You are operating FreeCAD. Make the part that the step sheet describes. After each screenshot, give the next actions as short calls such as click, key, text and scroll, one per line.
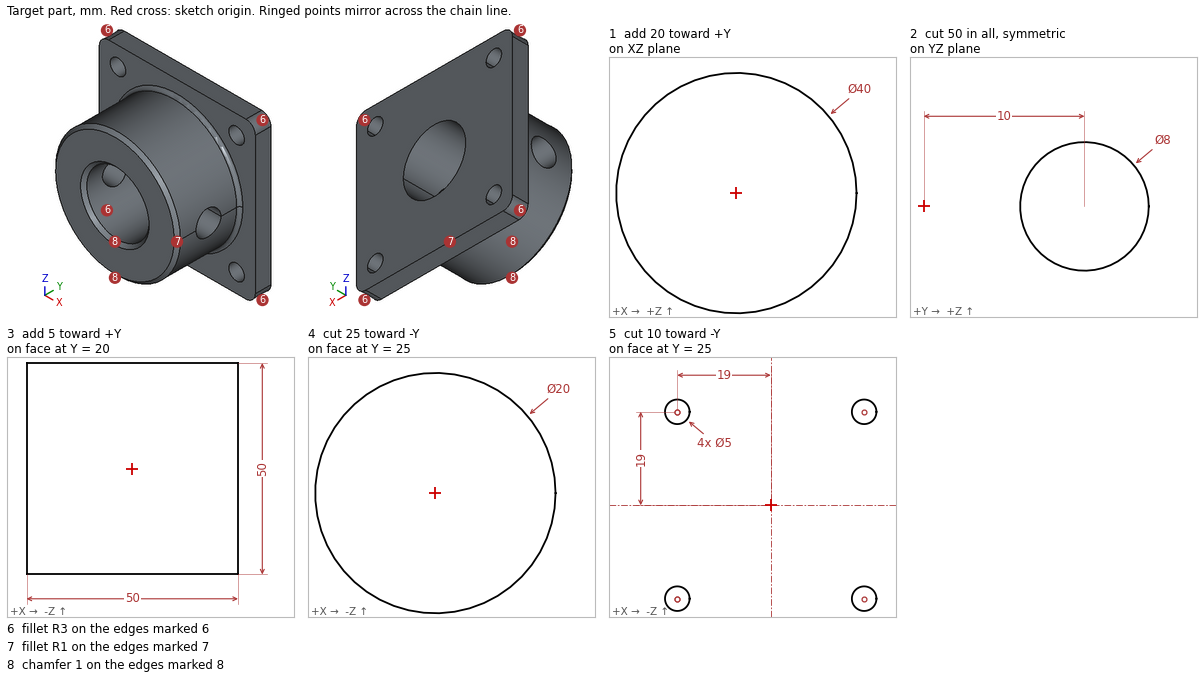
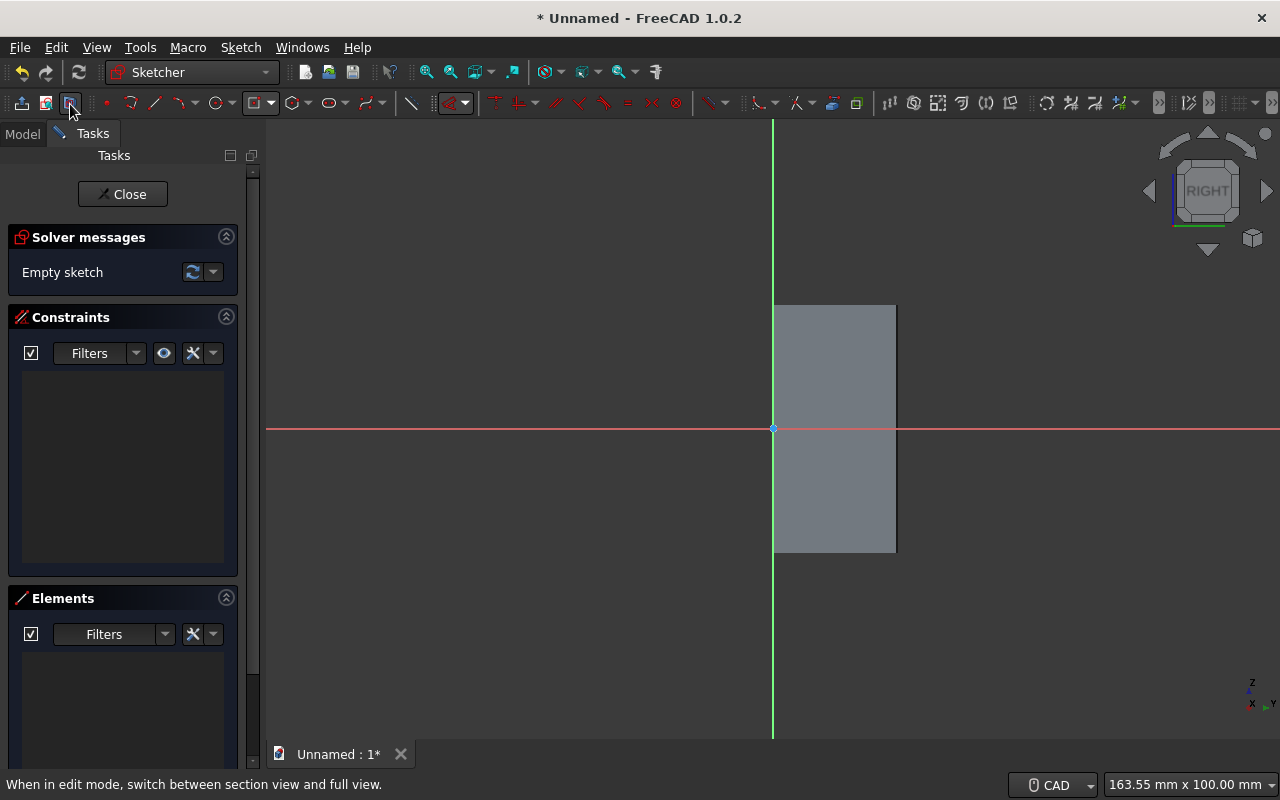
scroll(839, 429, up, 9)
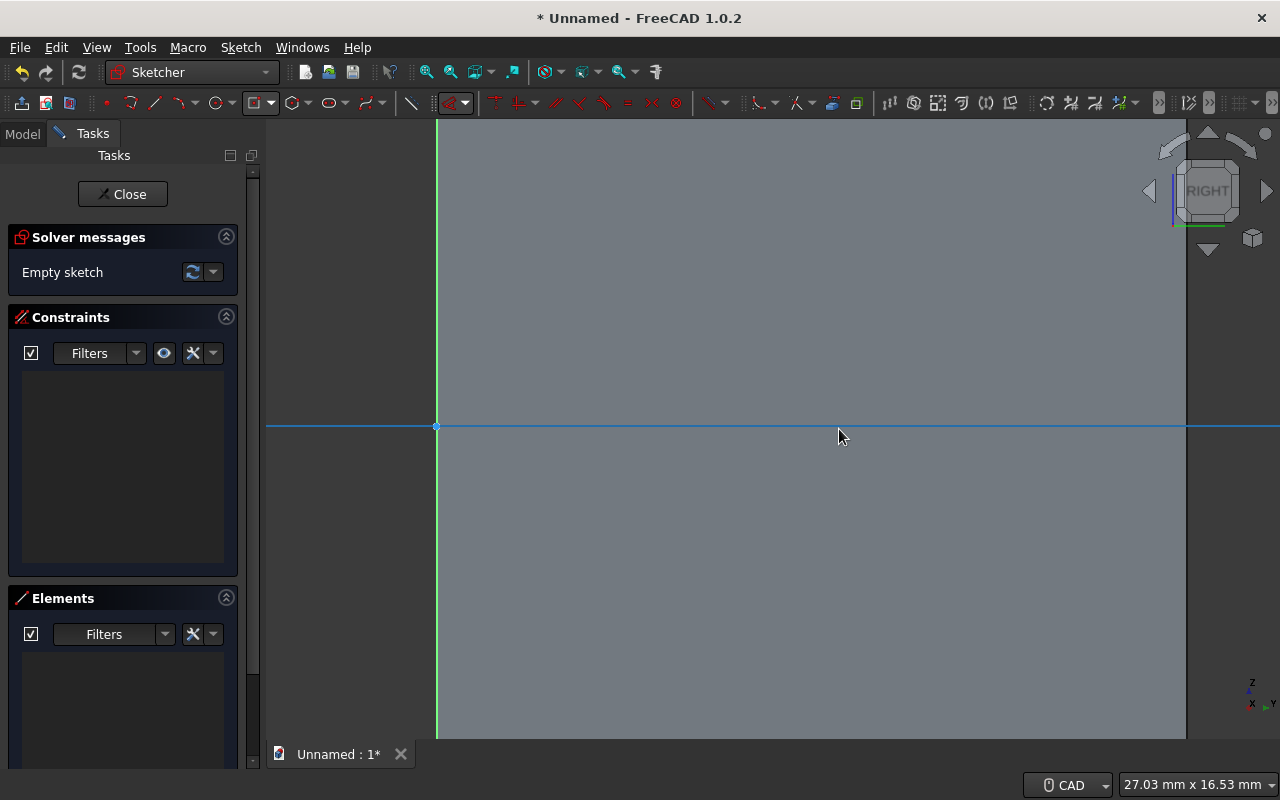
click(216, 104)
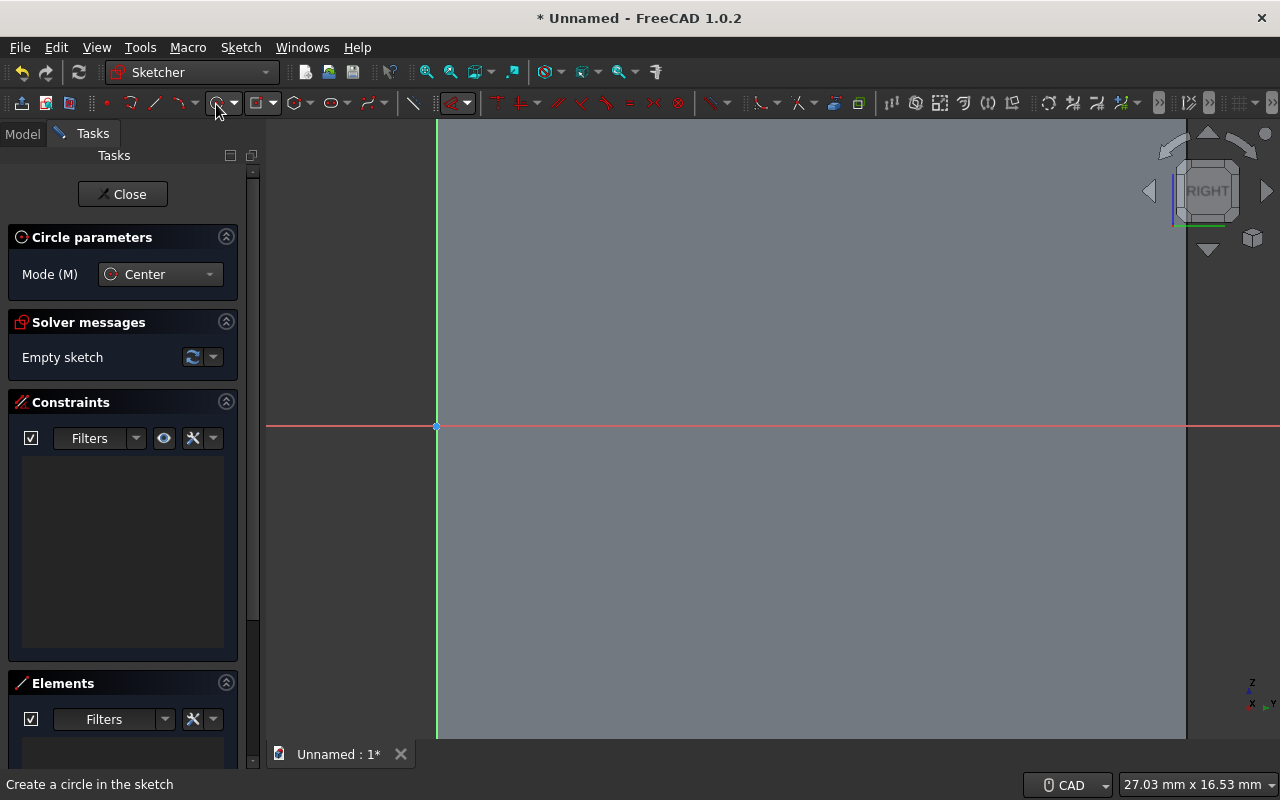
click(812, 426)
click(918, 320)
key(Escape)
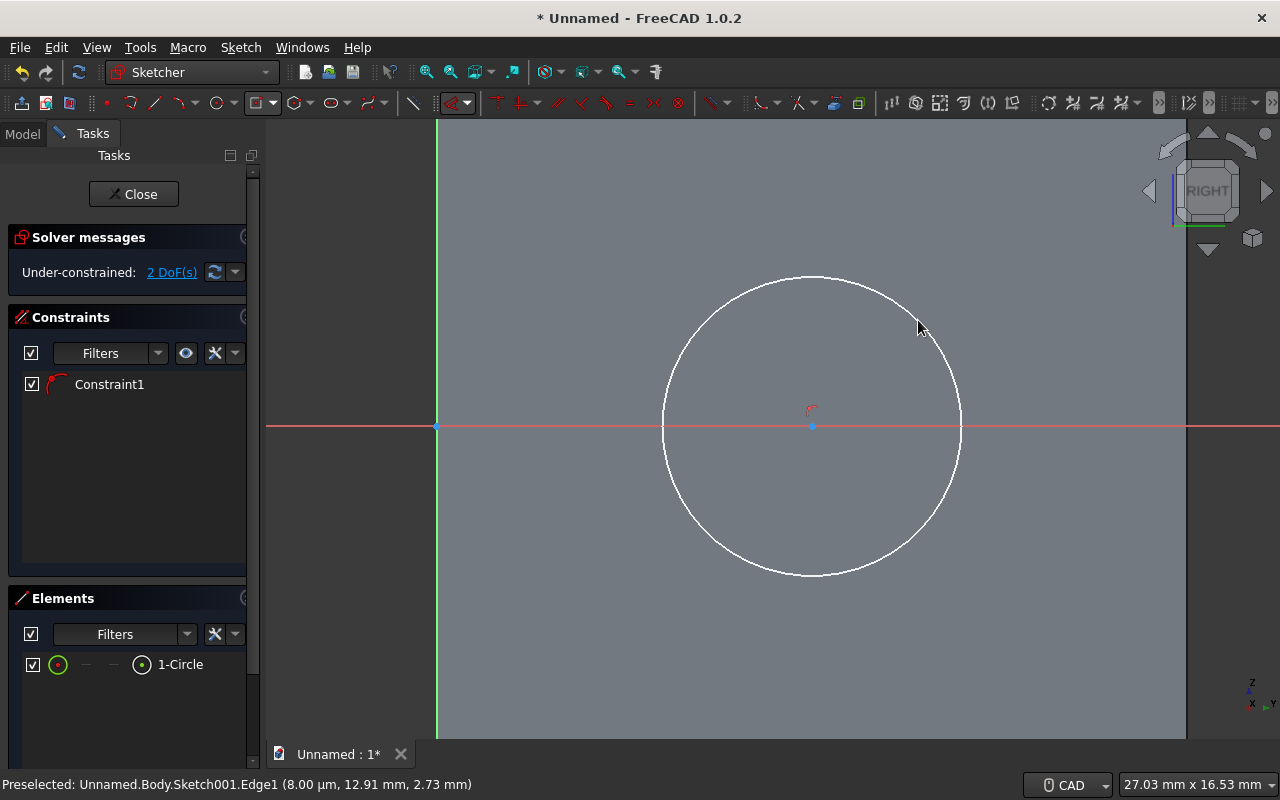
click(917, 320)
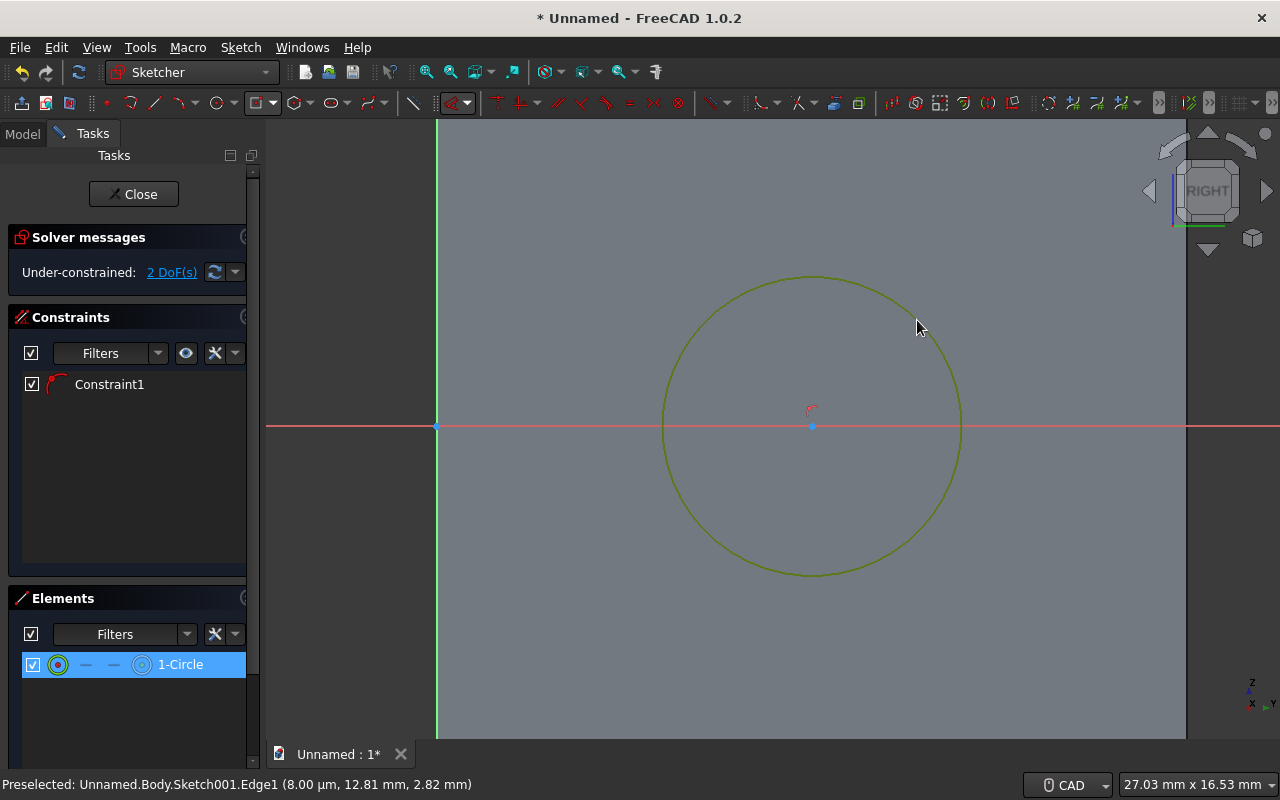
key(k)
key(o)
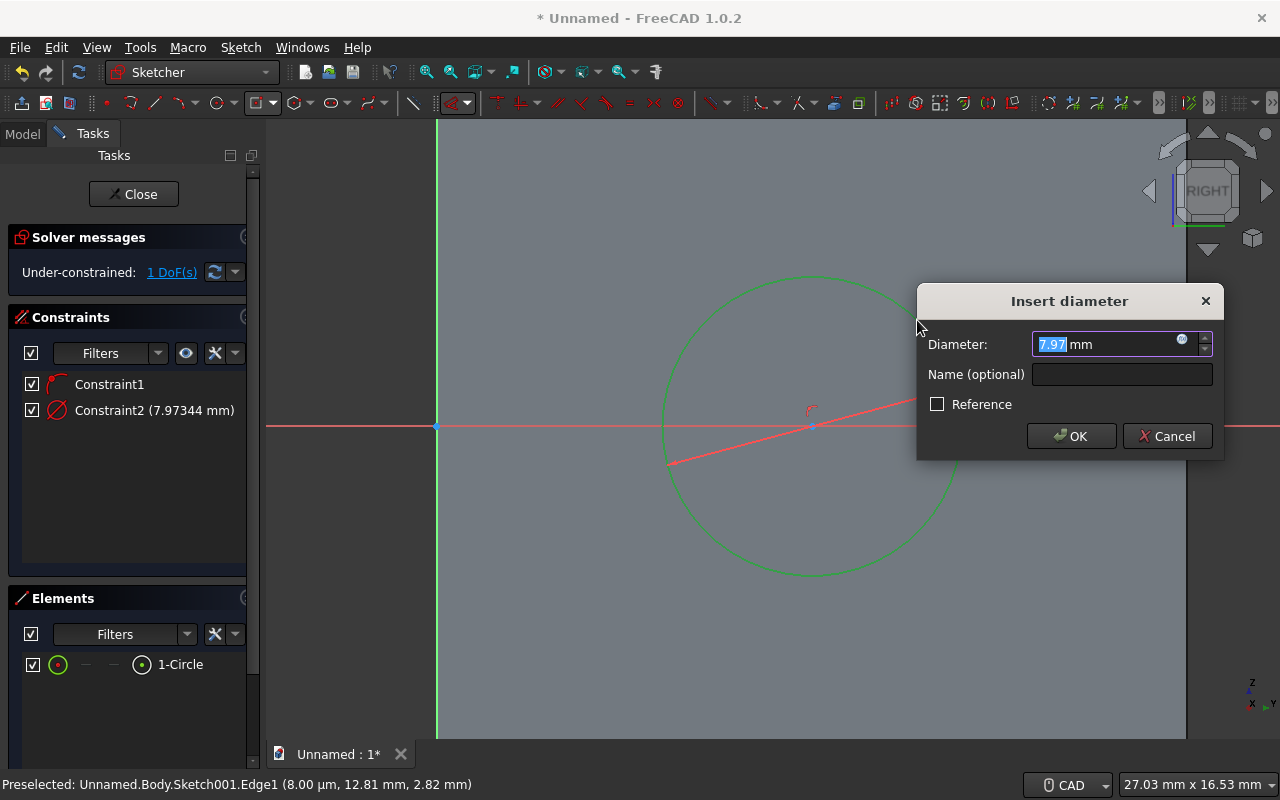
text(8)
key(Return)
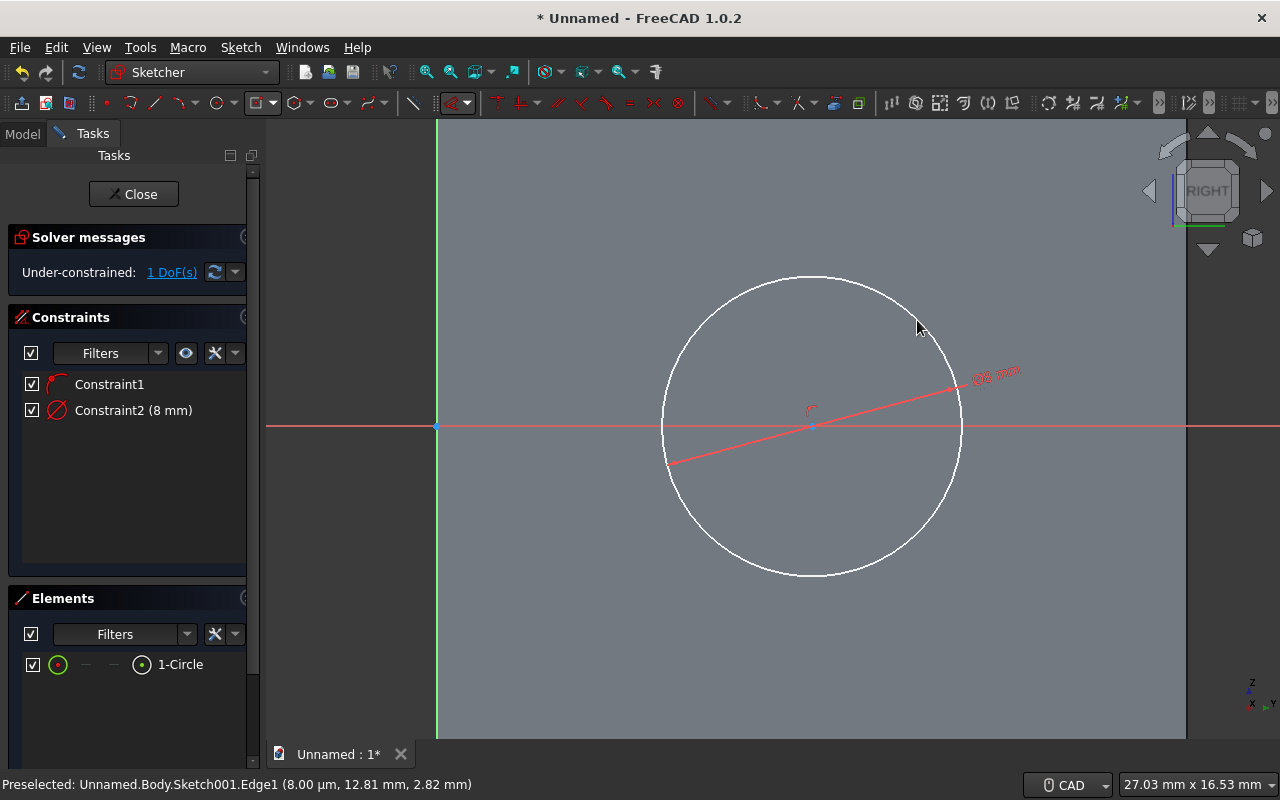
click(812, 426)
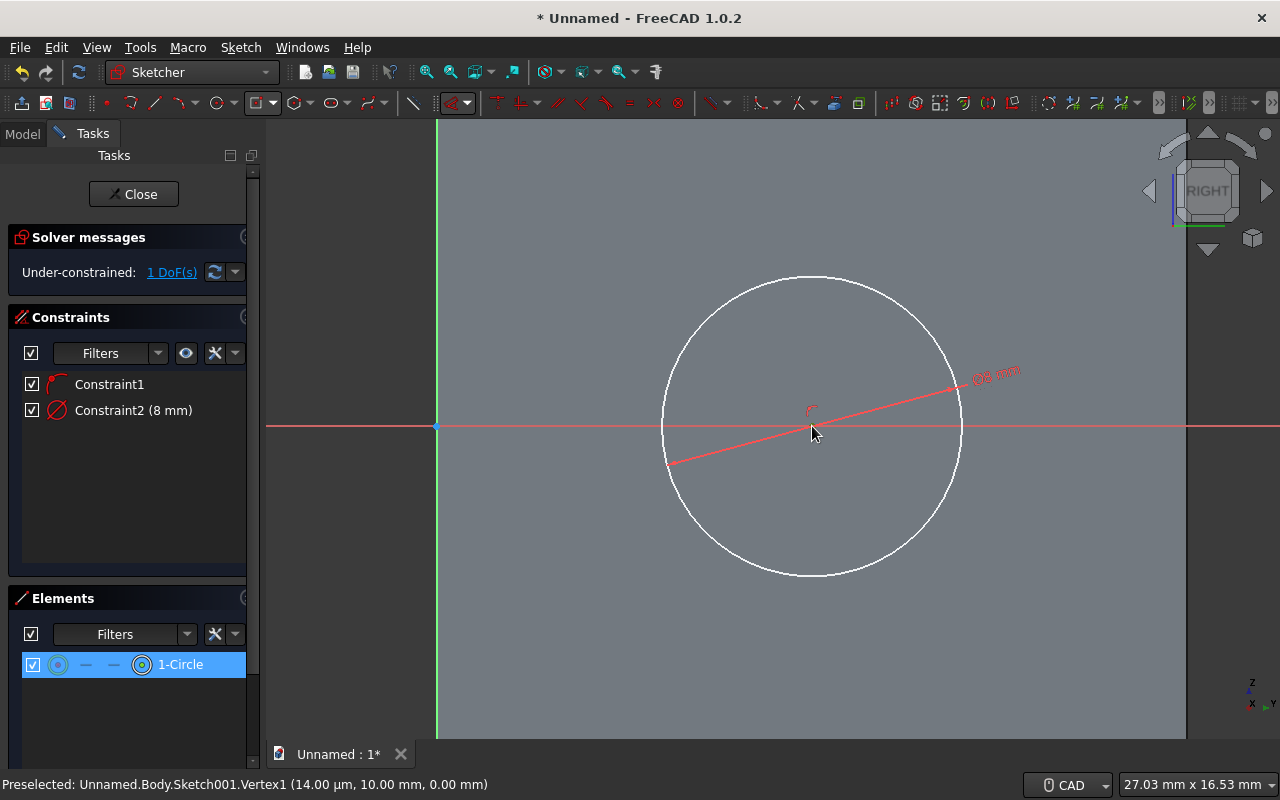
click(470, 104)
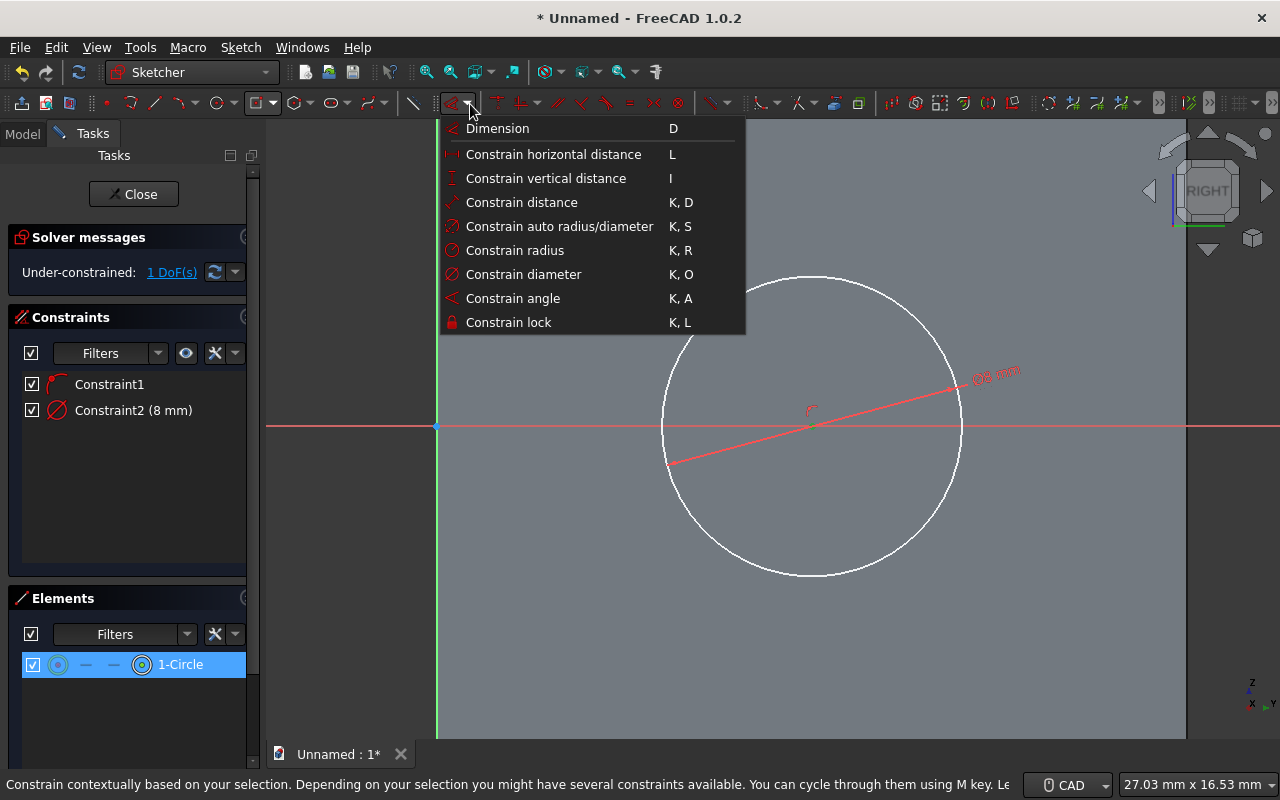
click(593, 154)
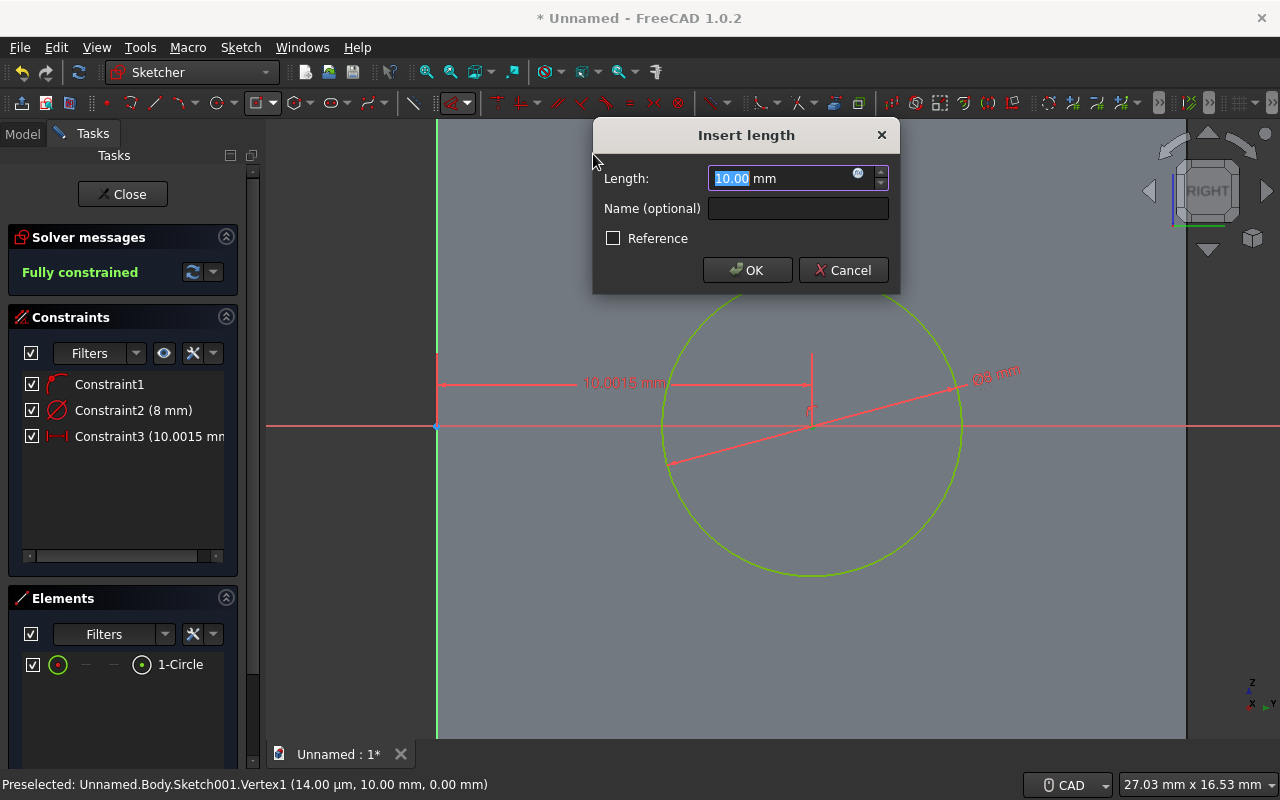
text(10)
key(Return)